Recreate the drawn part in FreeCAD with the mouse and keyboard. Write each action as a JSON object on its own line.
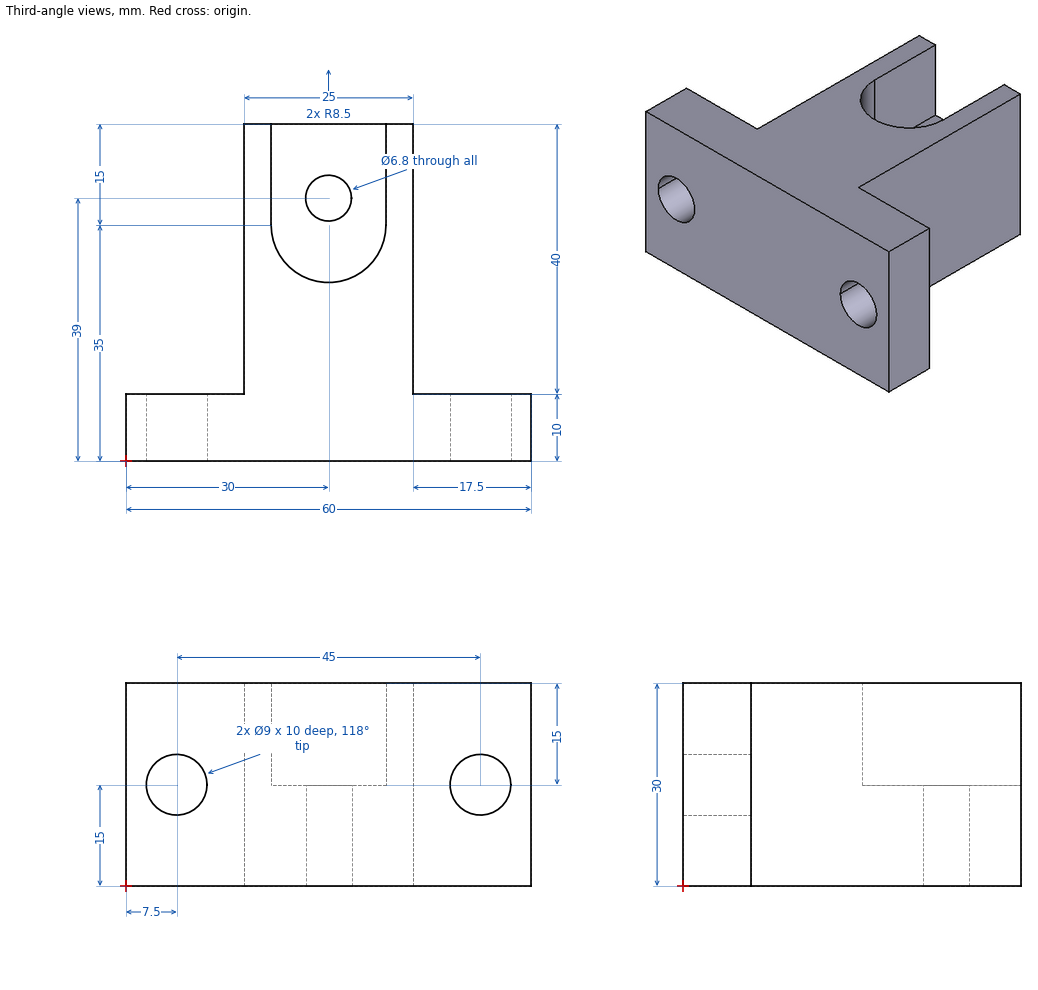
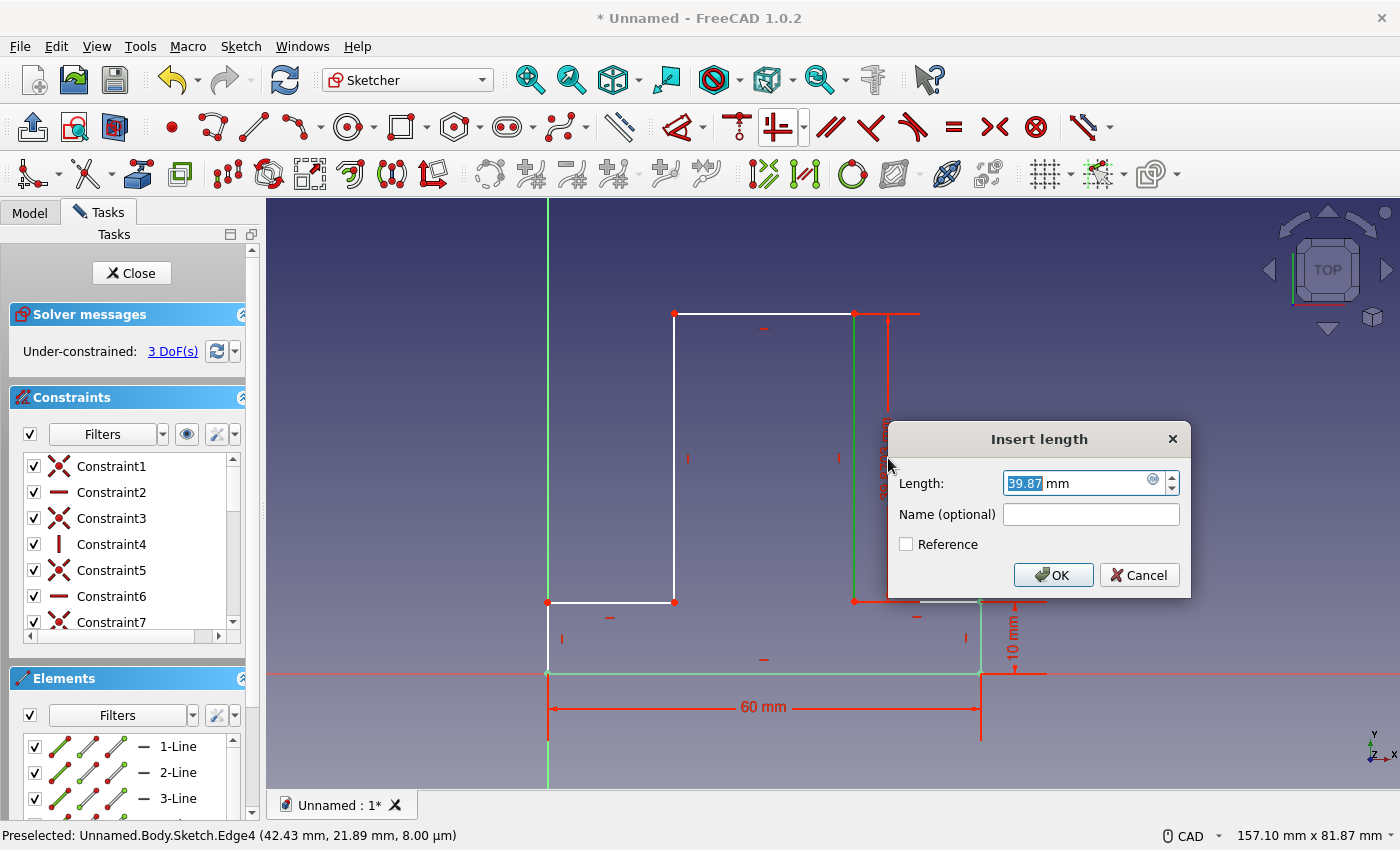
{"action": "type", "text": "40"}
{"action": "key", "text": "Return"}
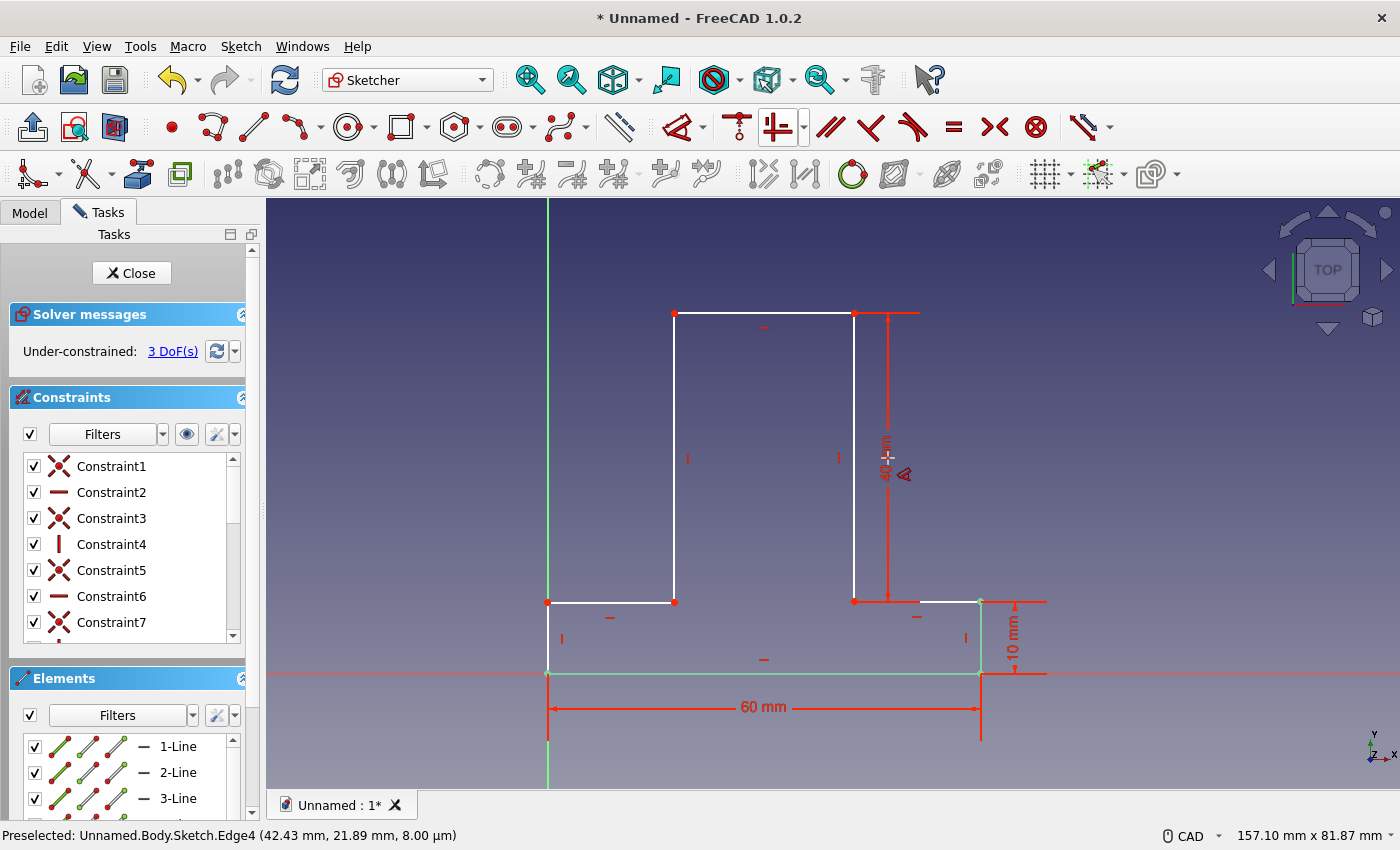
{"action": "left_click", "coordinate": [800, 313]}
{"action": "left_click", "coordinate": [764, 279]}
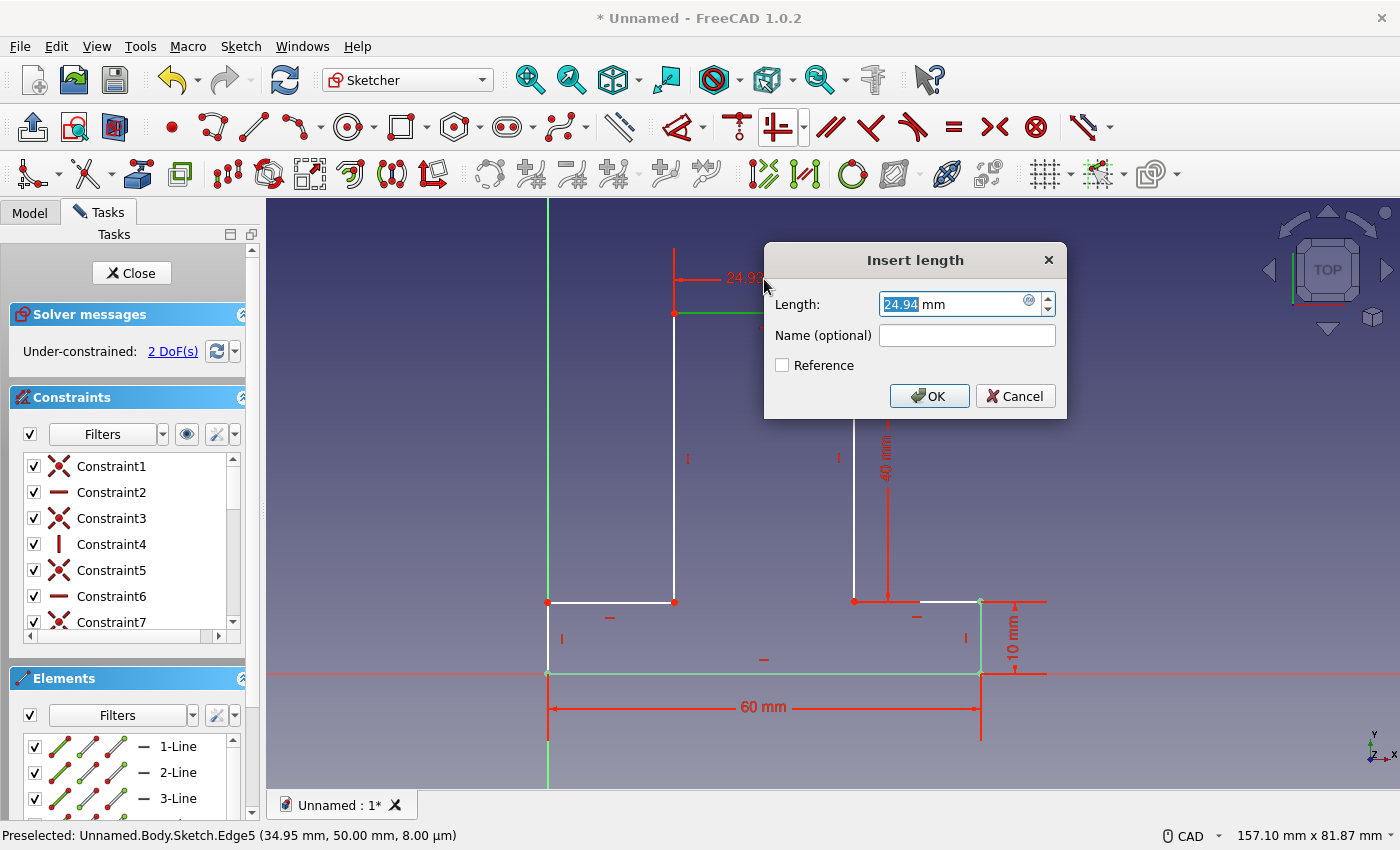
{"action": "type", "text": "25"}
{"action": "key", "text": "Return"}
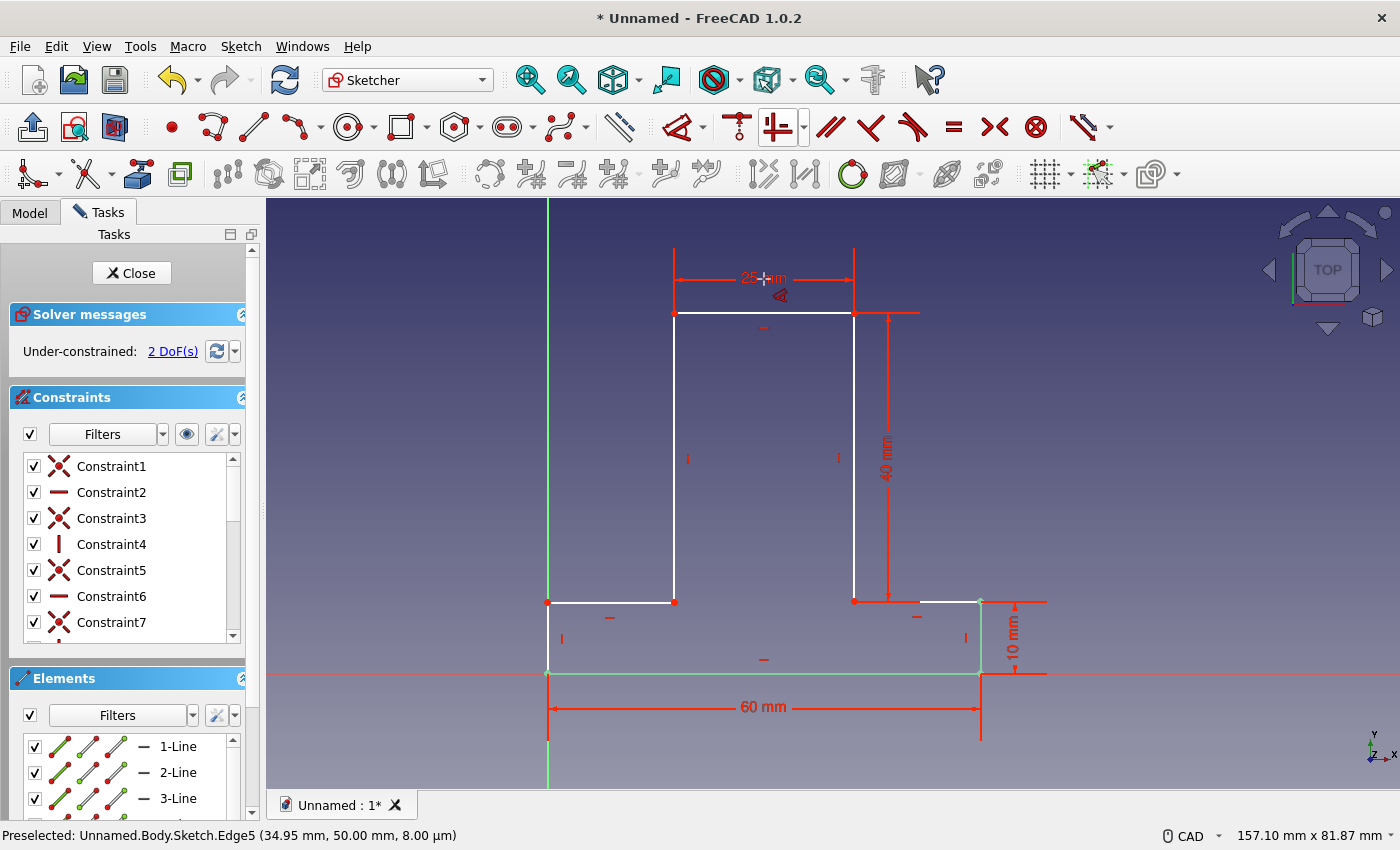
{"action": "left_click", "coordinate": [674, 400]}
{"action": "left_click", "coordinate": [640, 458]}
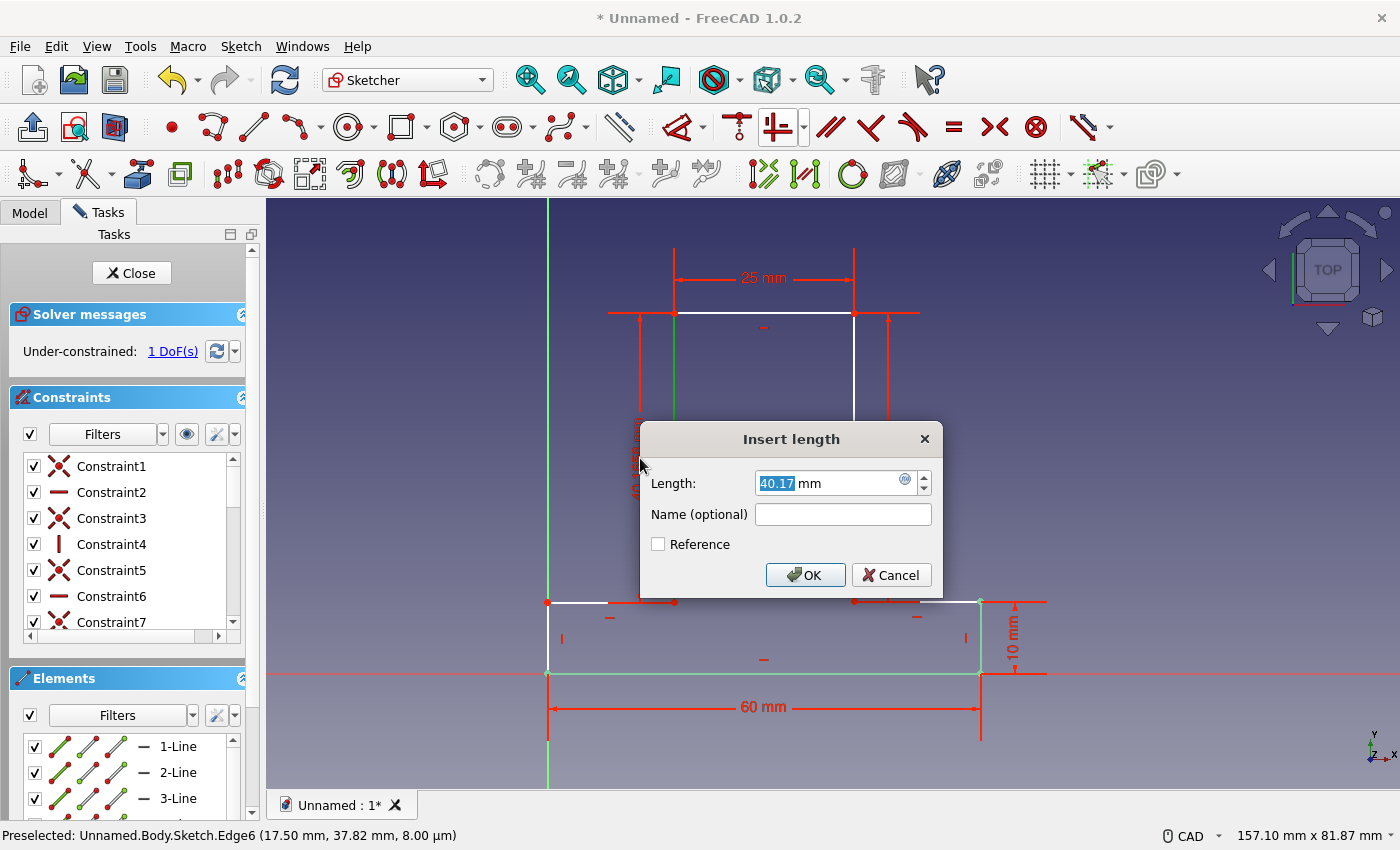
{"action": "type", "text": "40"}
{"action": "key", "text": "Return"}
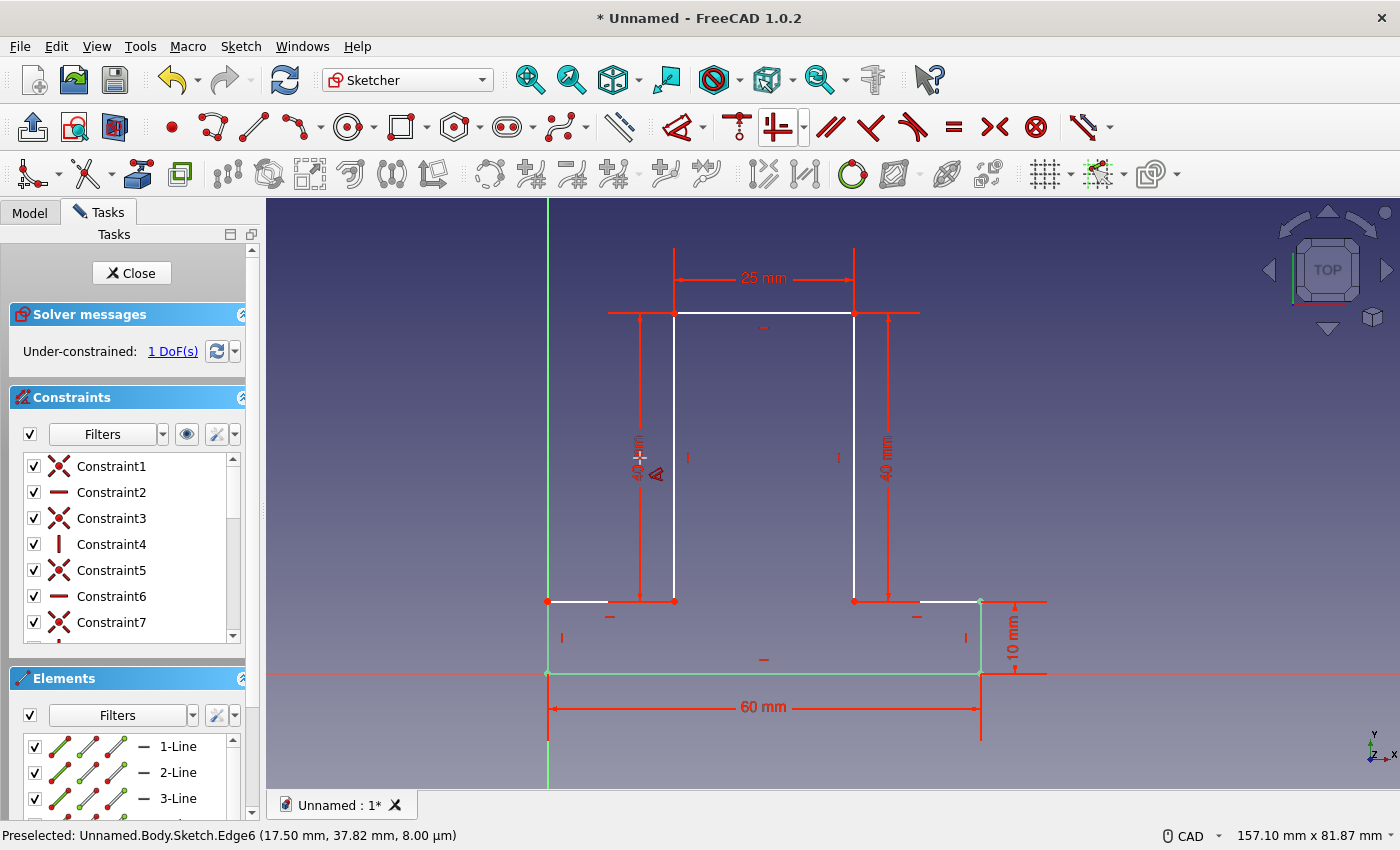
{"action": "left_click", "coordinate": [943, 602]}
{"action": "left_click", "coordinate": [918, 636]}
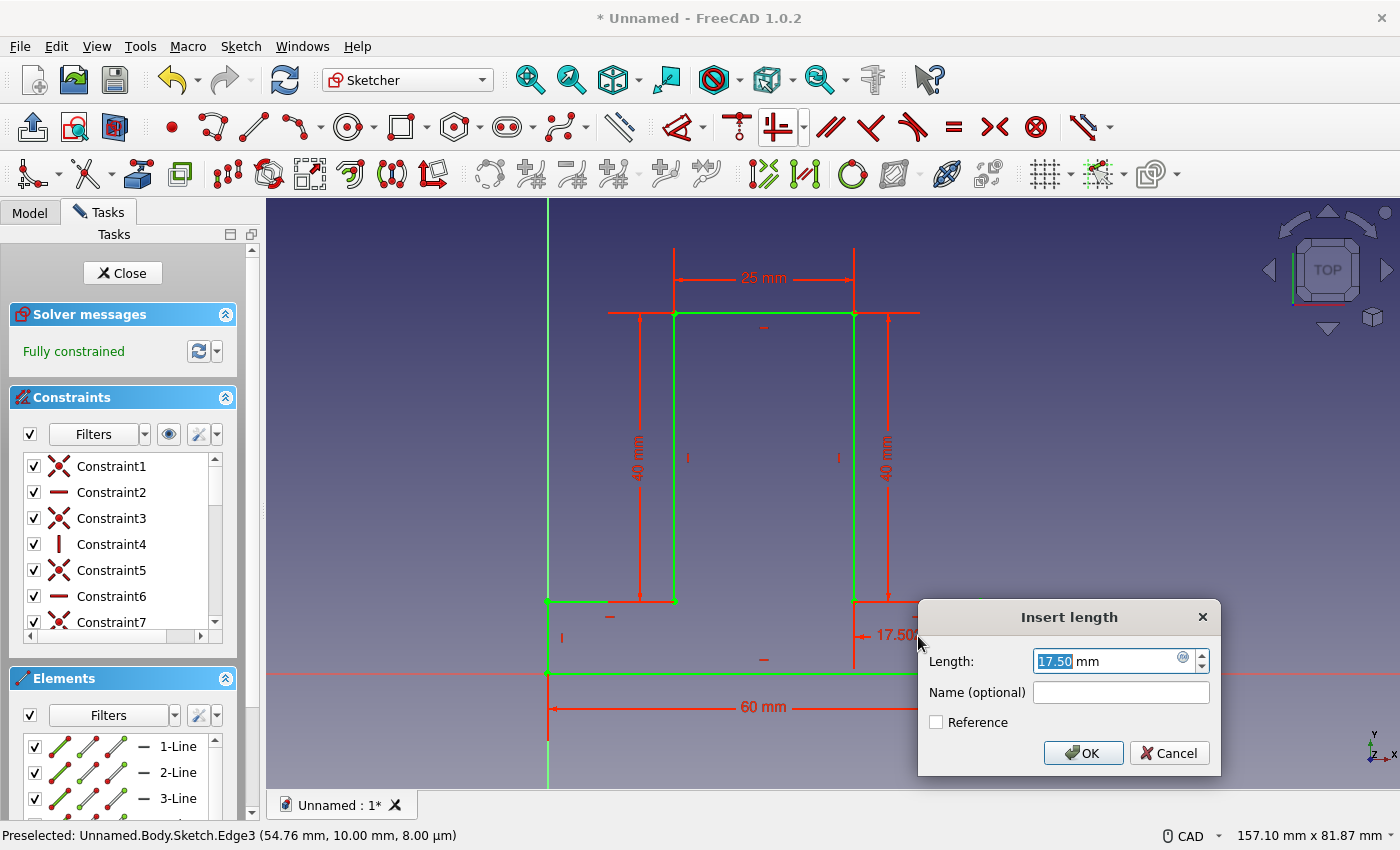
{"action": "type", "text": "17.5"}
{"action": "key", "text": "Return"}
{"action": "key", "text": "Escape"}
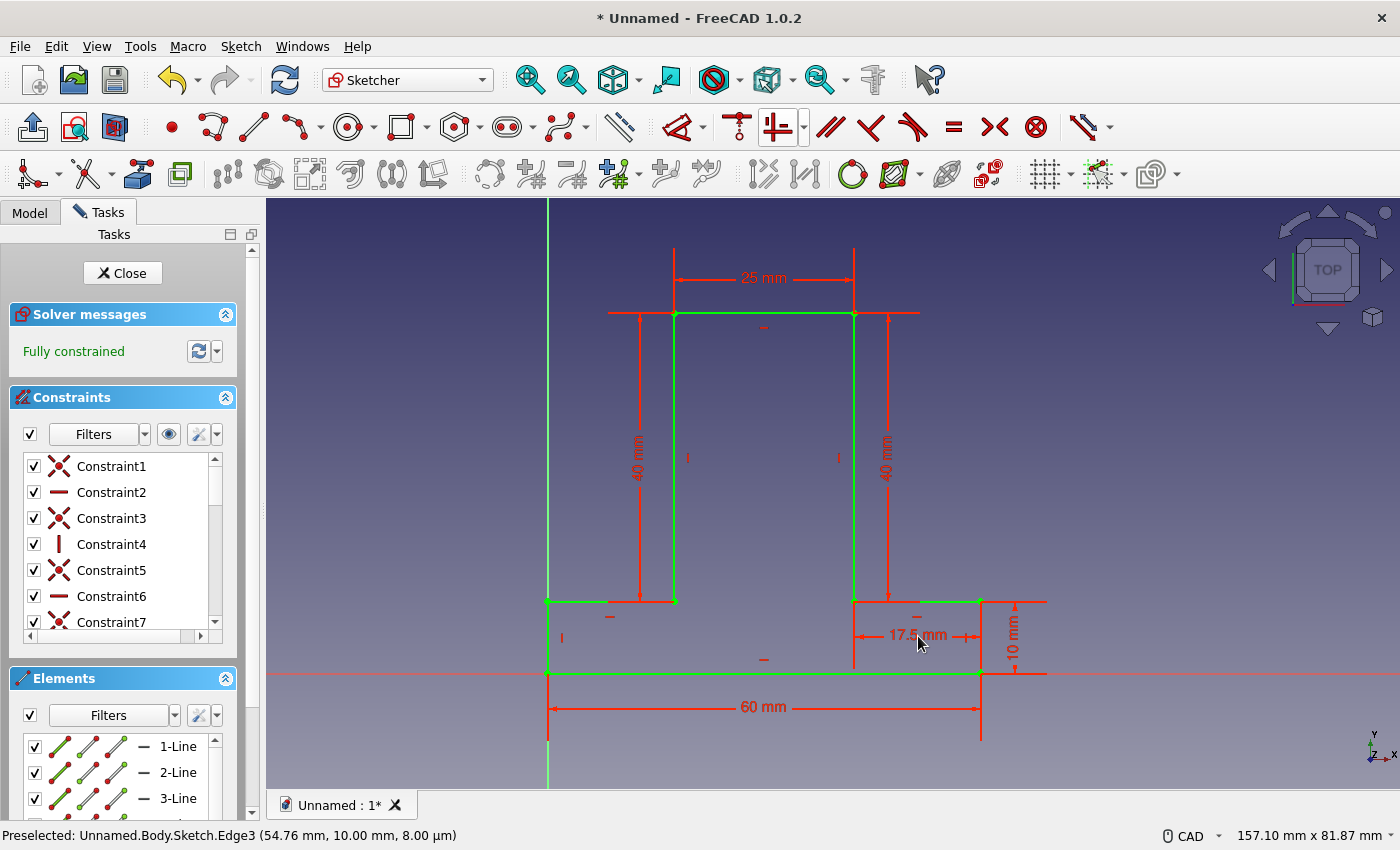
{"action": "left_click", "coordinate": [123, 273]}